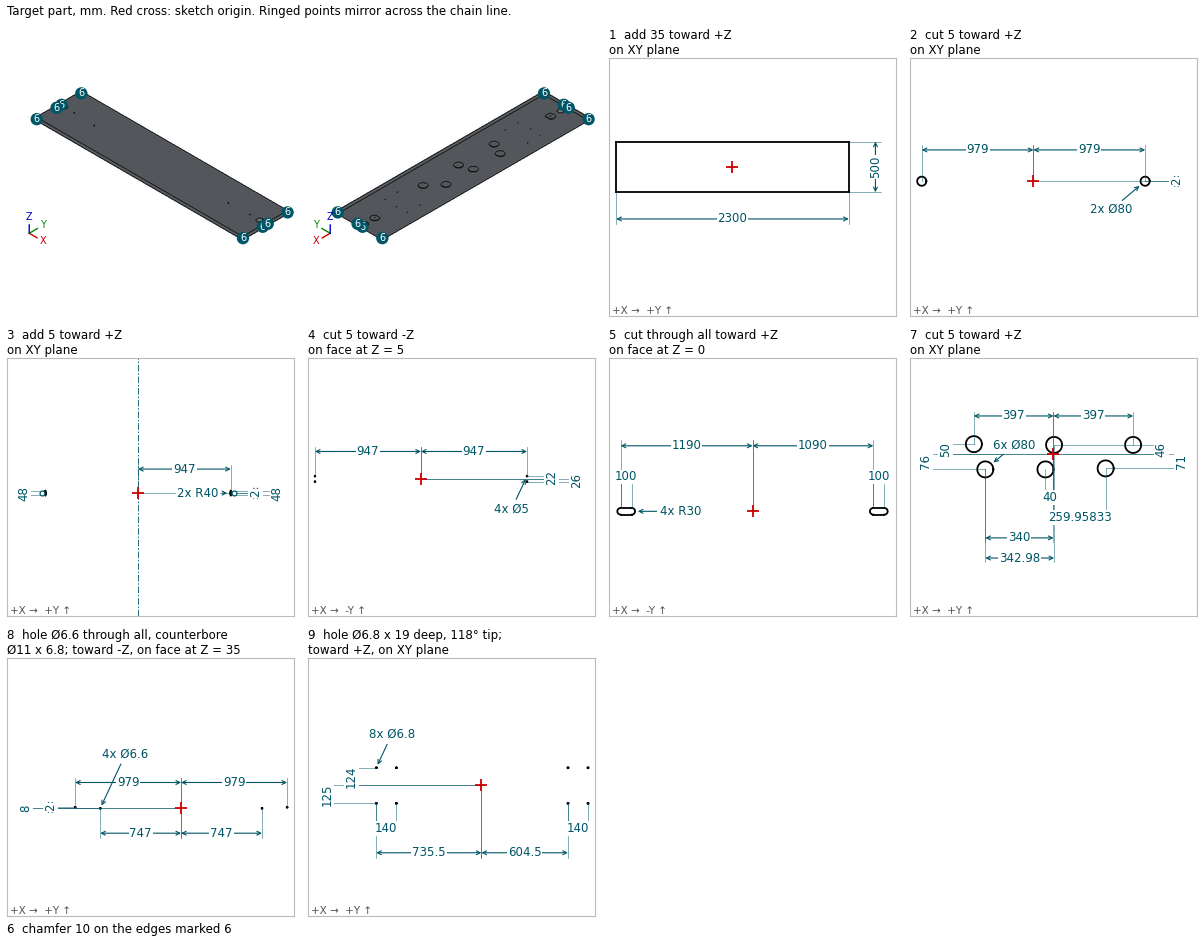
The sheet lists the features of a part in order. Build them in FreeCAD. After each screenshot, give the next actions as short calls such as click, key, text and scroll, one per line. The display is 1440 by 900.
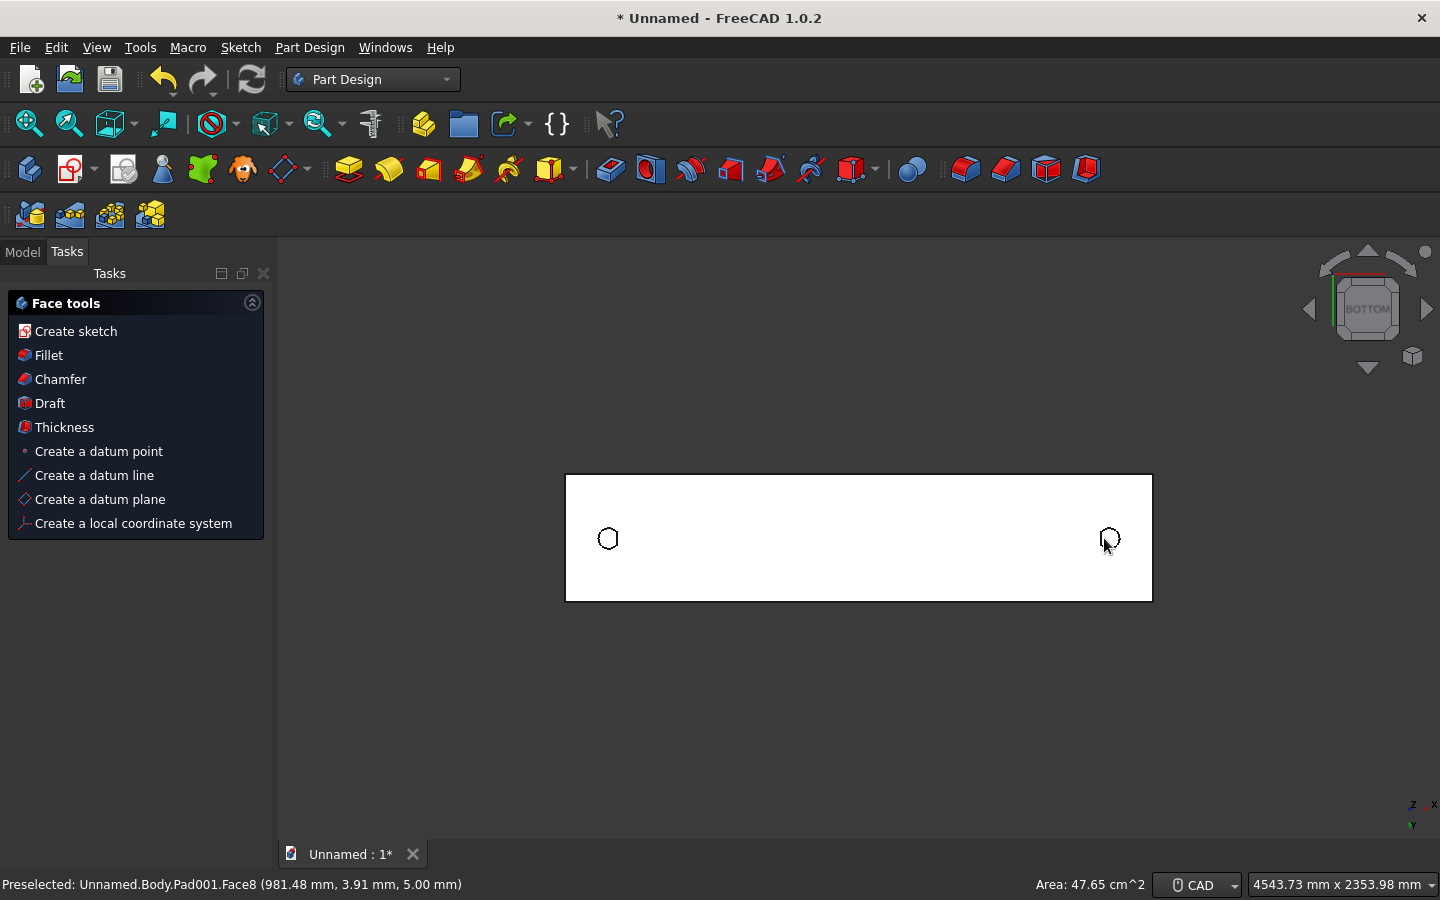
click(70, 170)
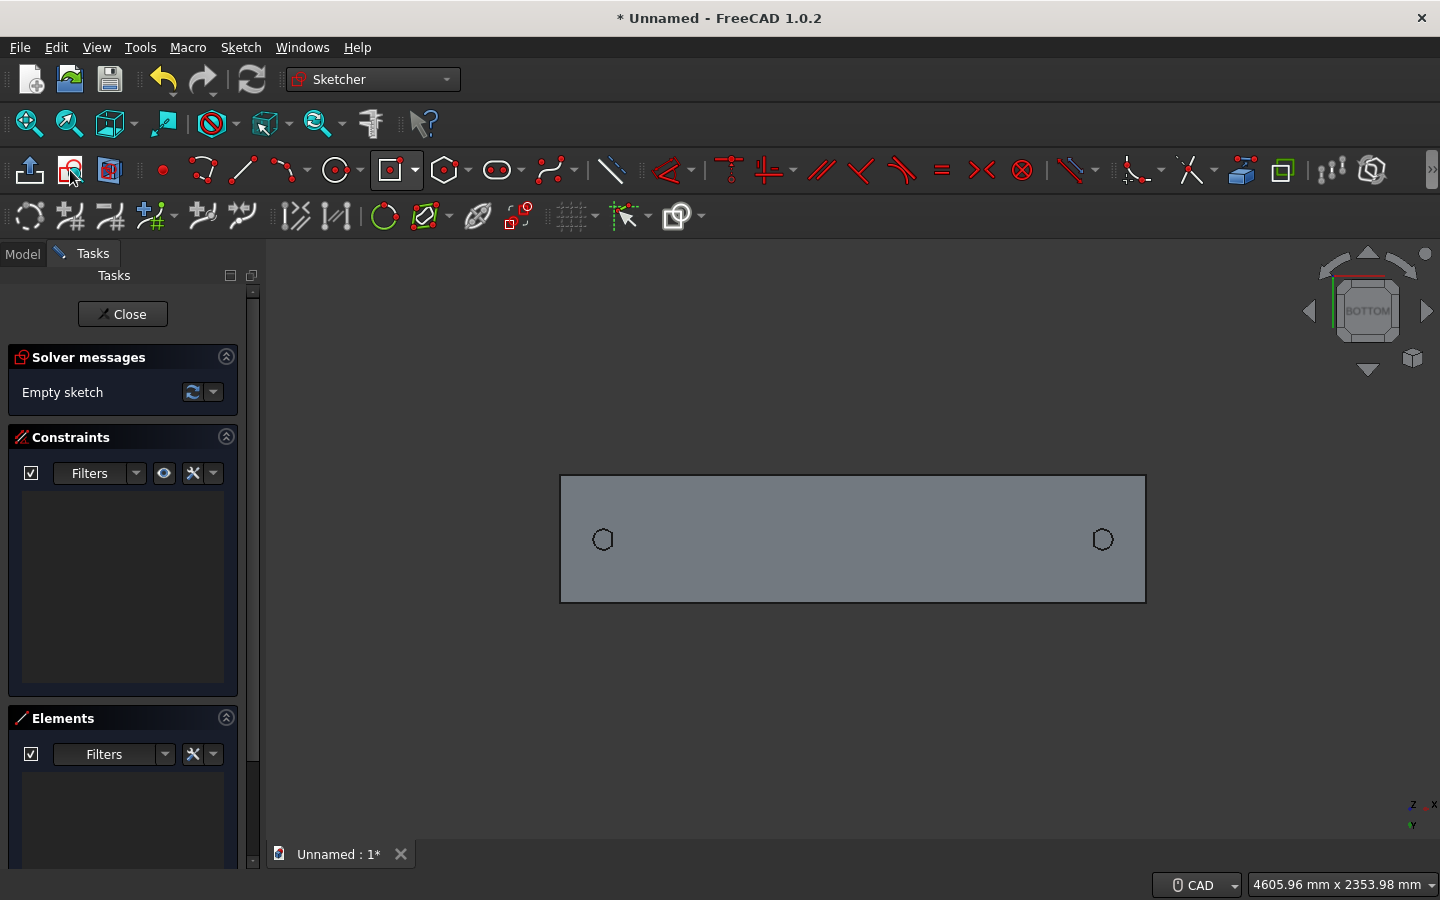
click(110, 170)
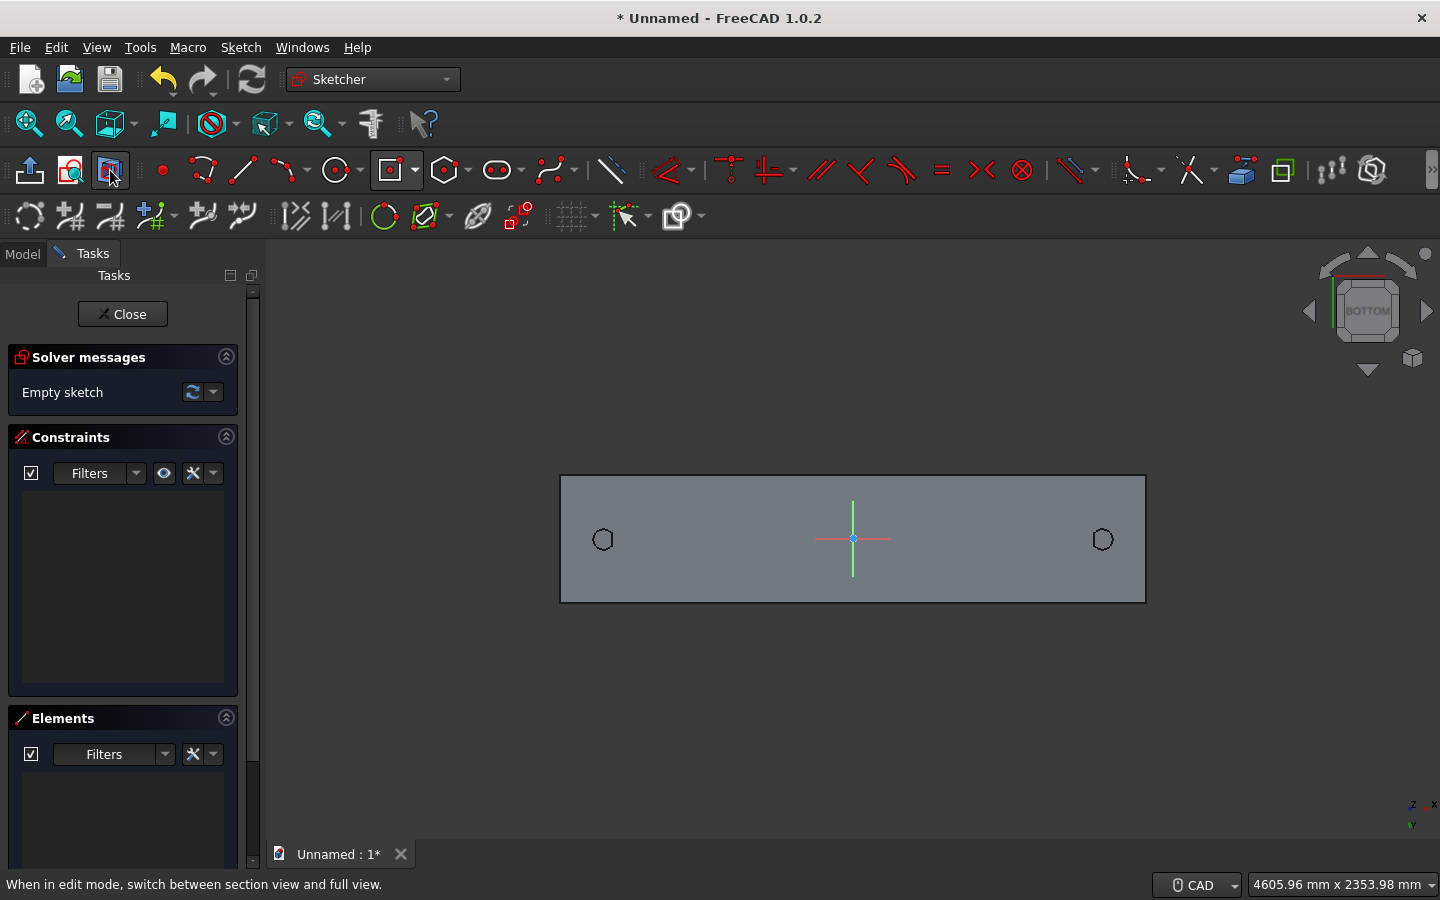
scroll(992, 541, up, 2)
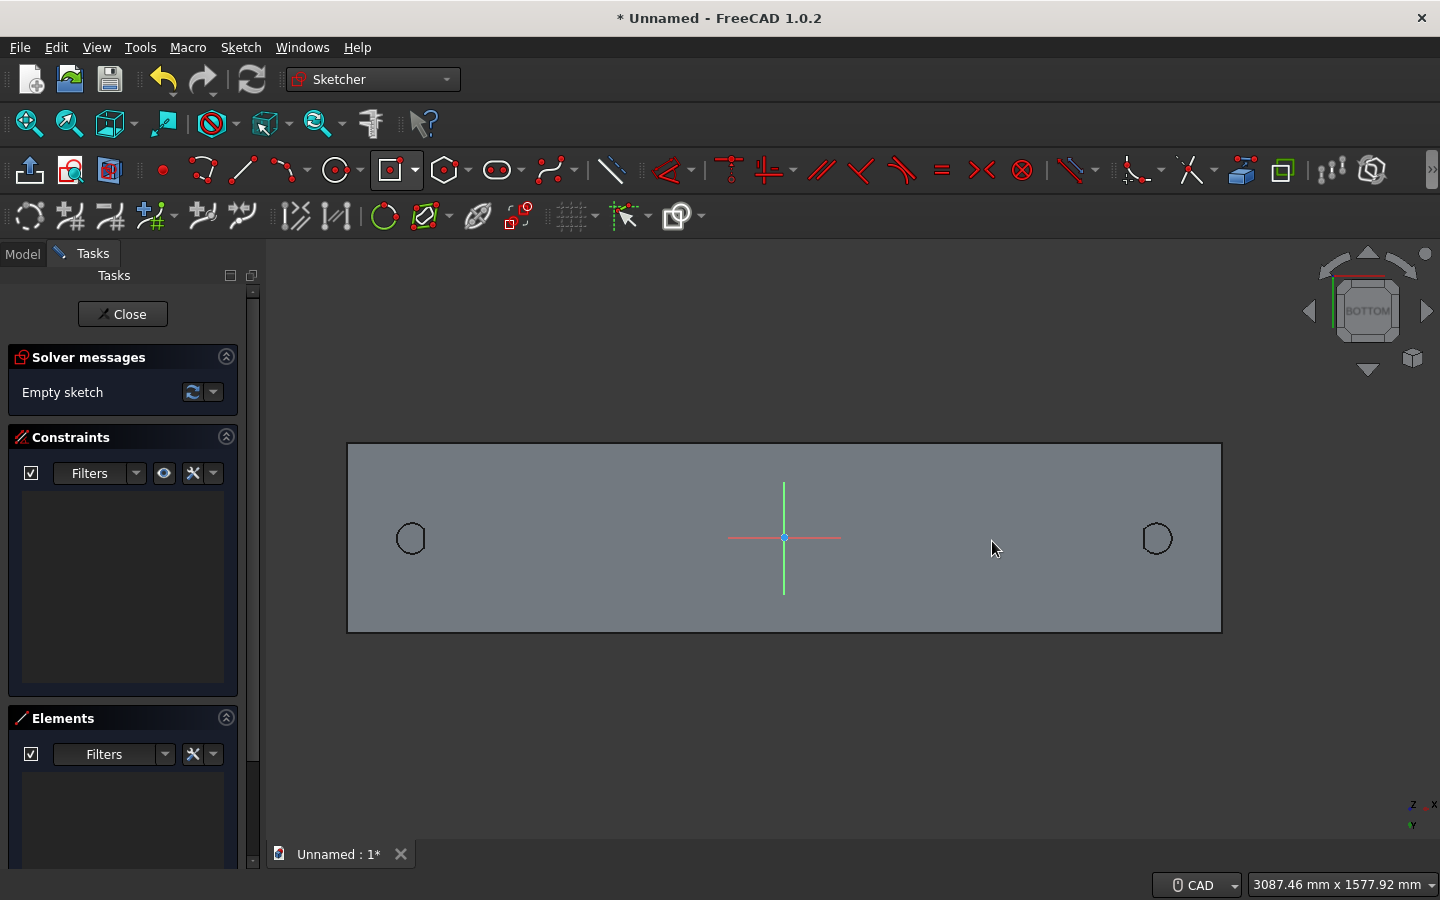
click(336, 170)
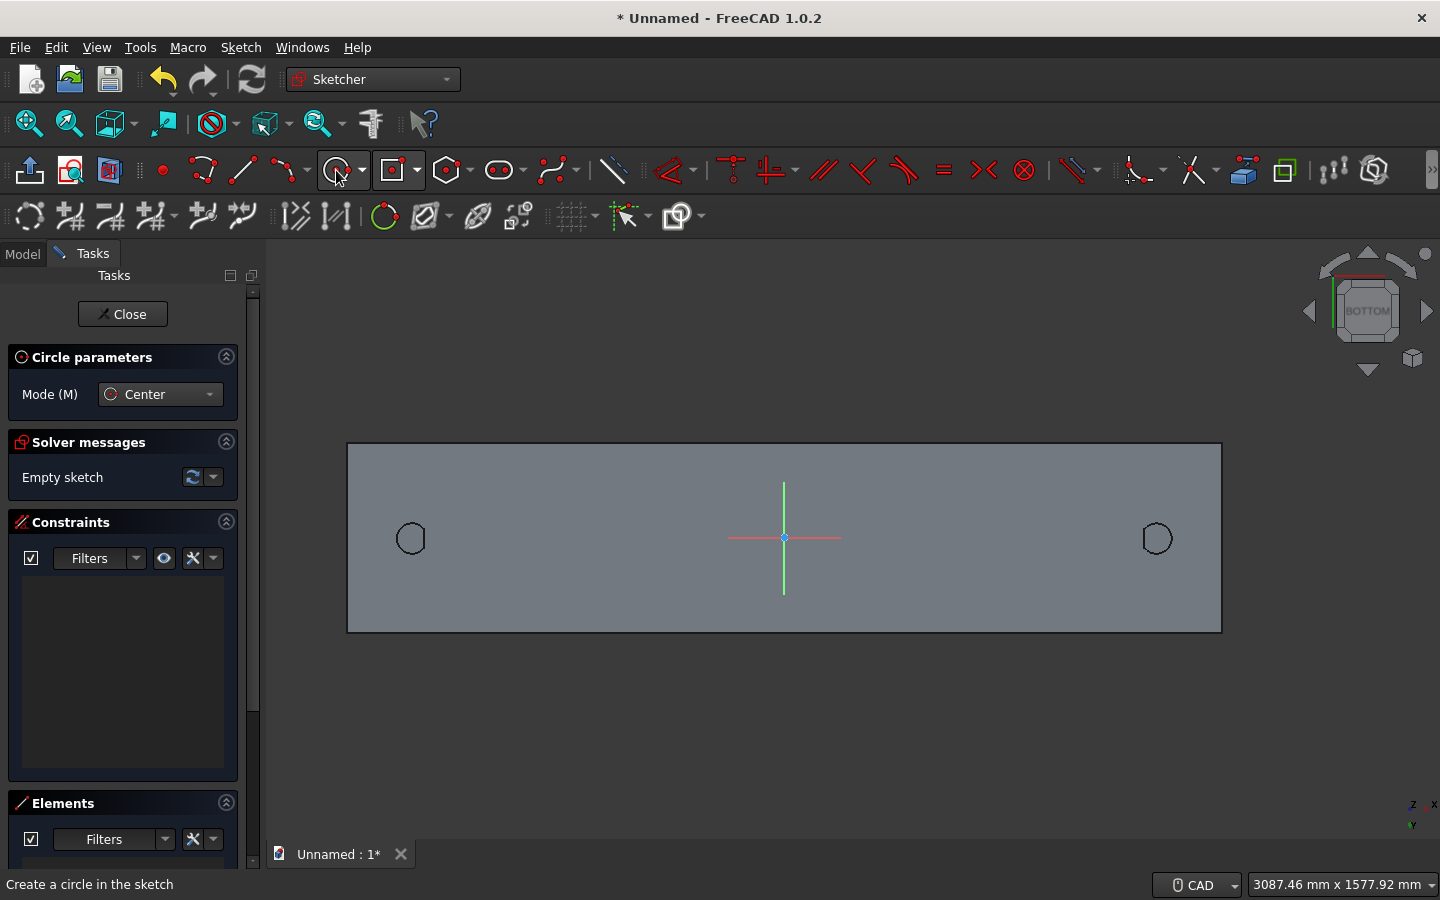
scroll(1144, 529, up, 16)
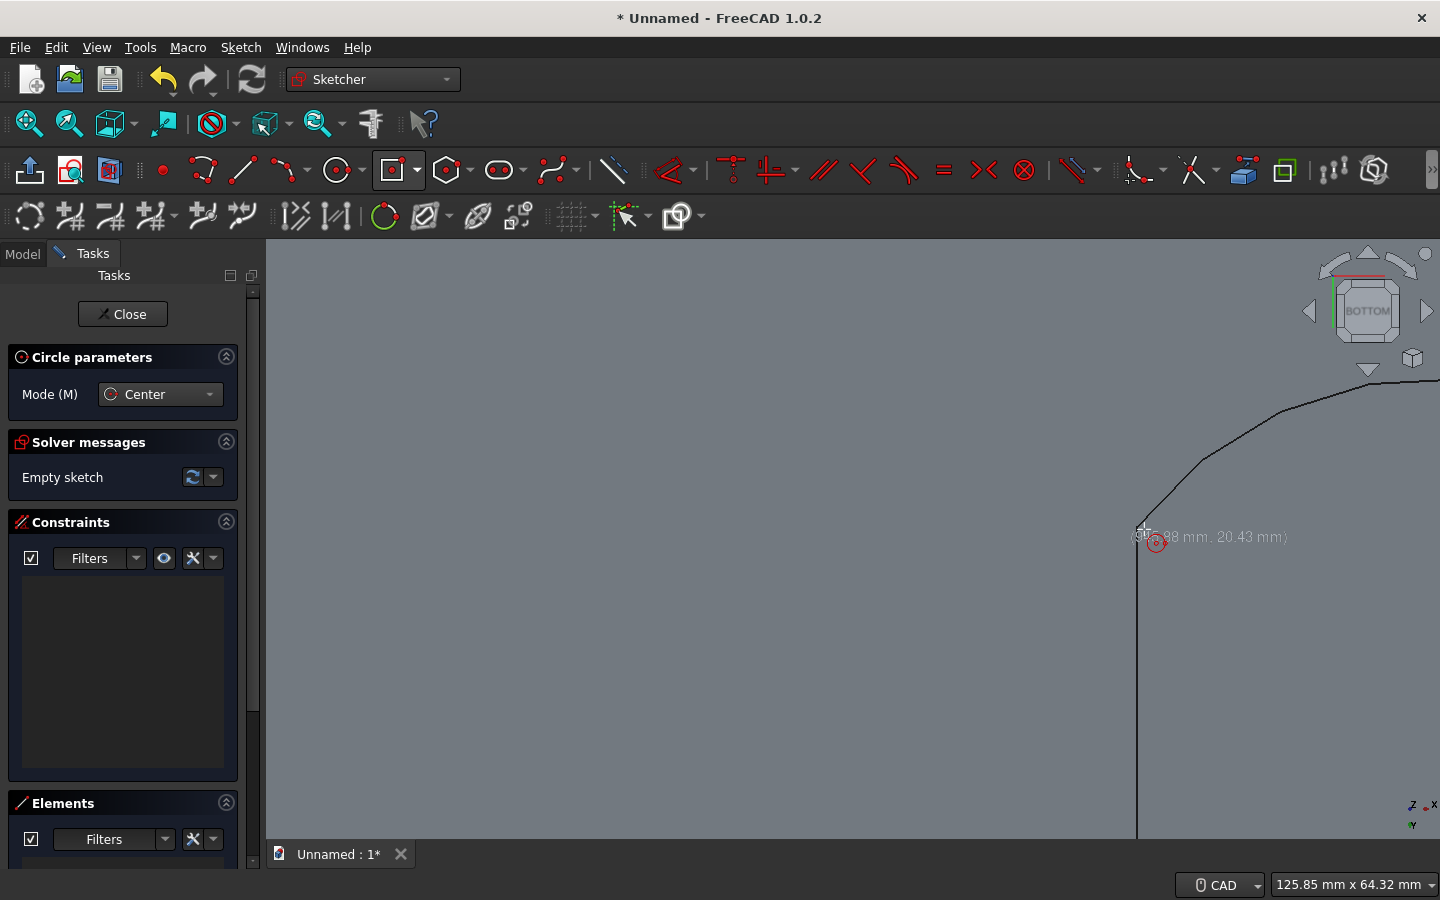
scroll(1229, 528, down, 15)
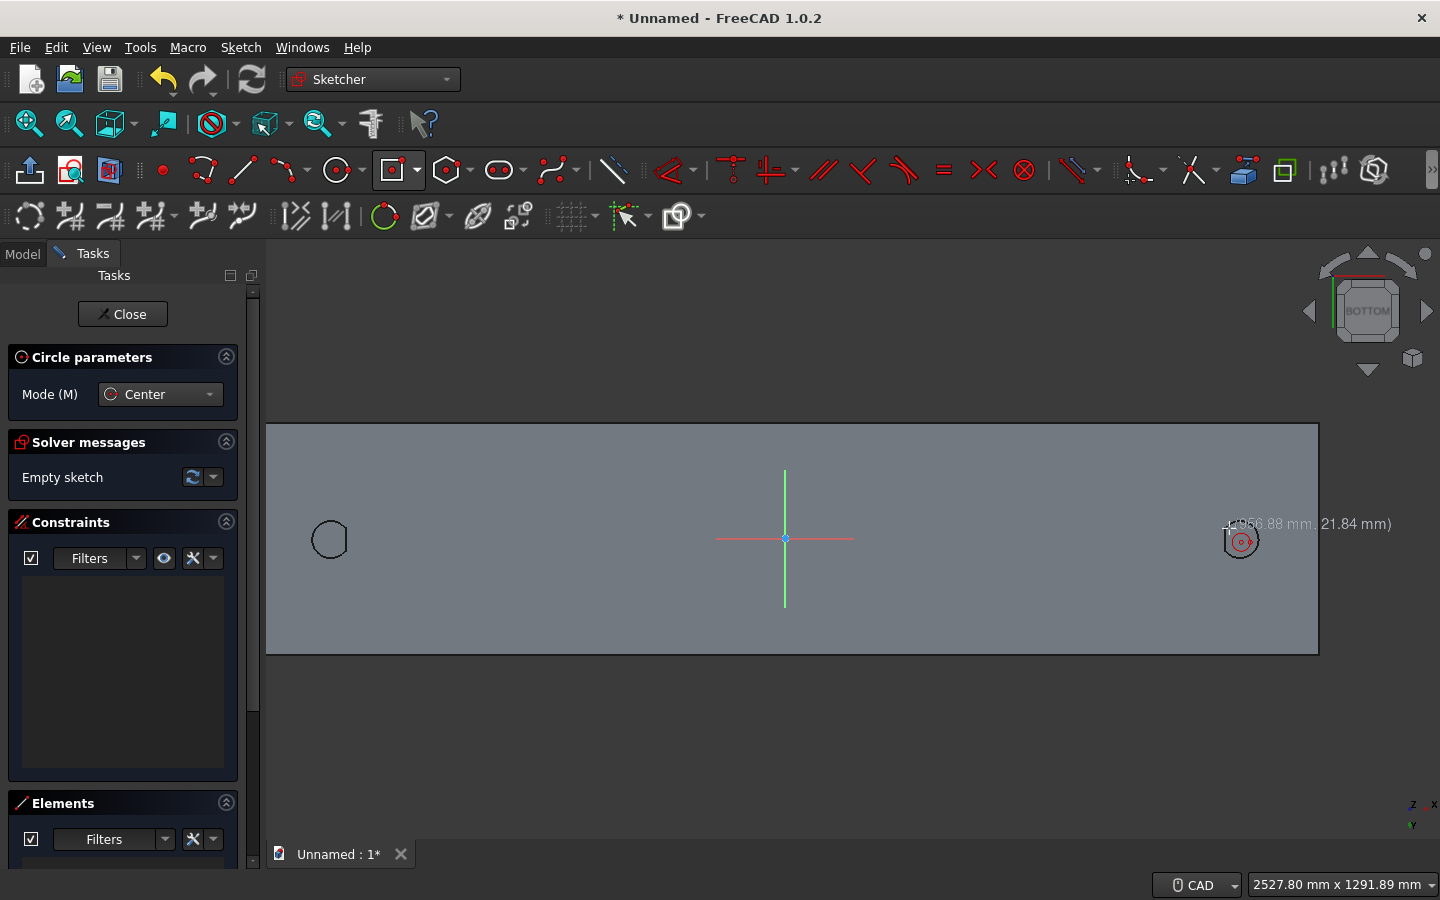
scroll(1225, 528, up, 3)